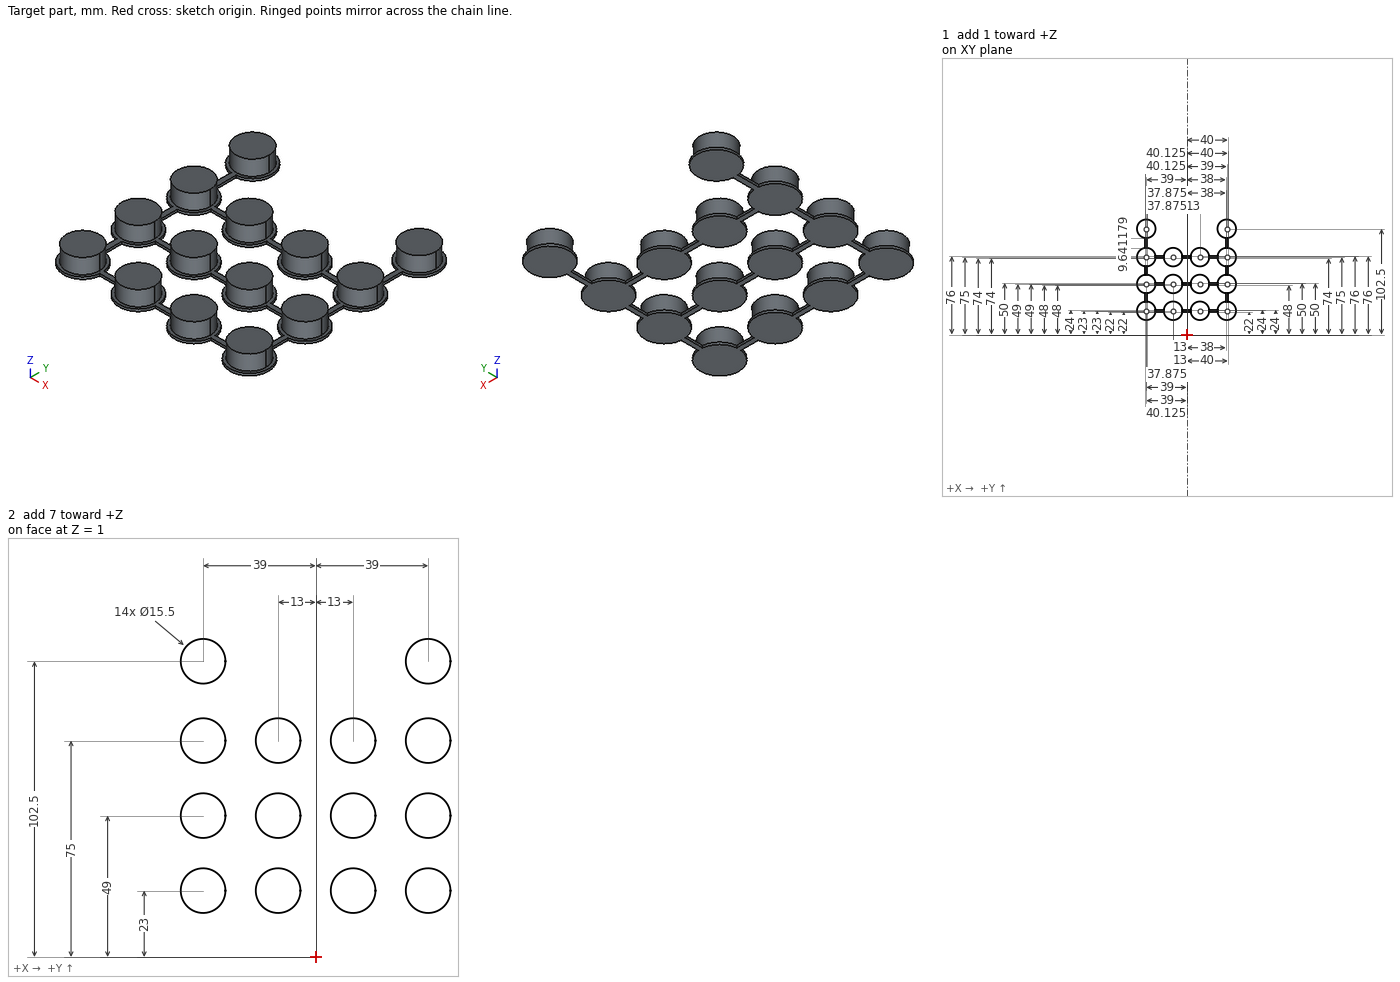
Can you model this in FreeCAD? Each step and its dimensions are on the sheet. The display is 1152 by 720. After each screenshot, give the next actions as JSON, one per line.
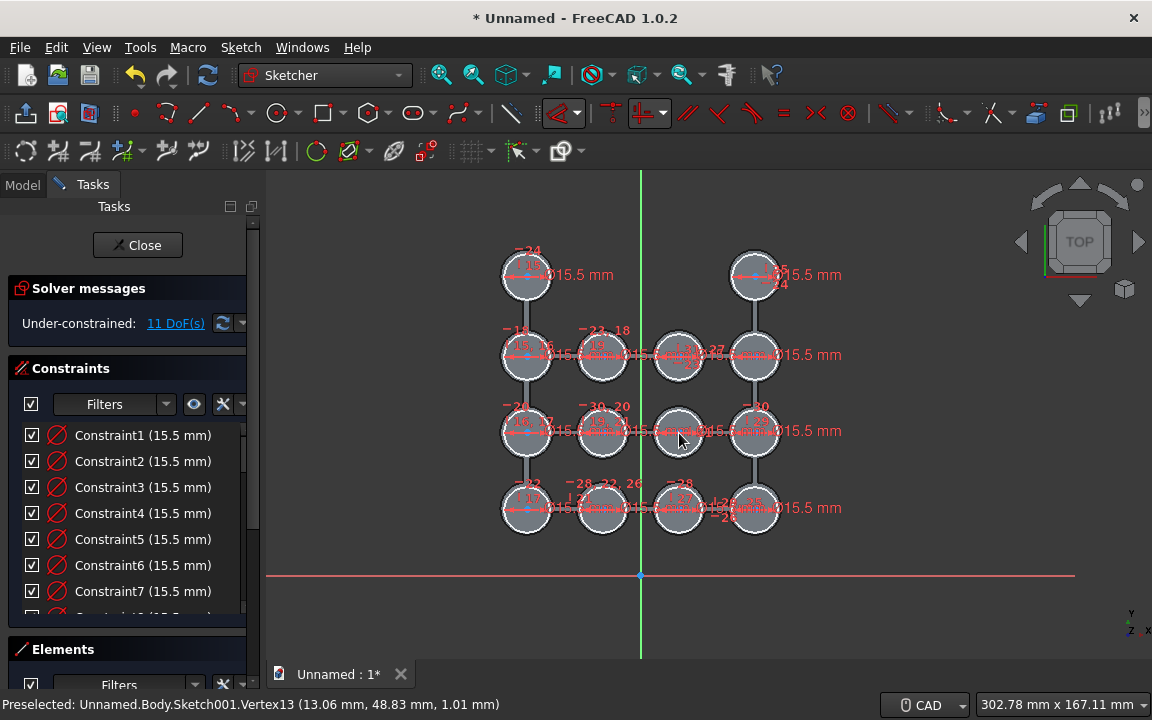
{"action": "left_click", "coordinate": [603, 433]}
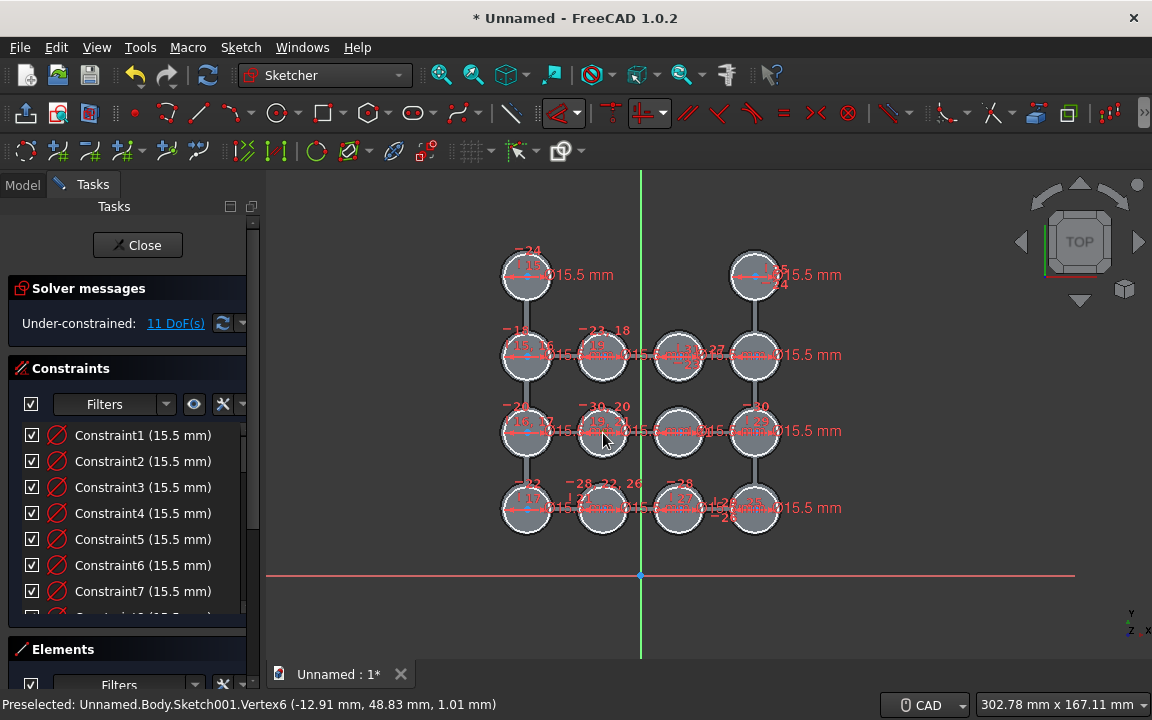
{"action": "left_click", "coordinate": [679, 433]}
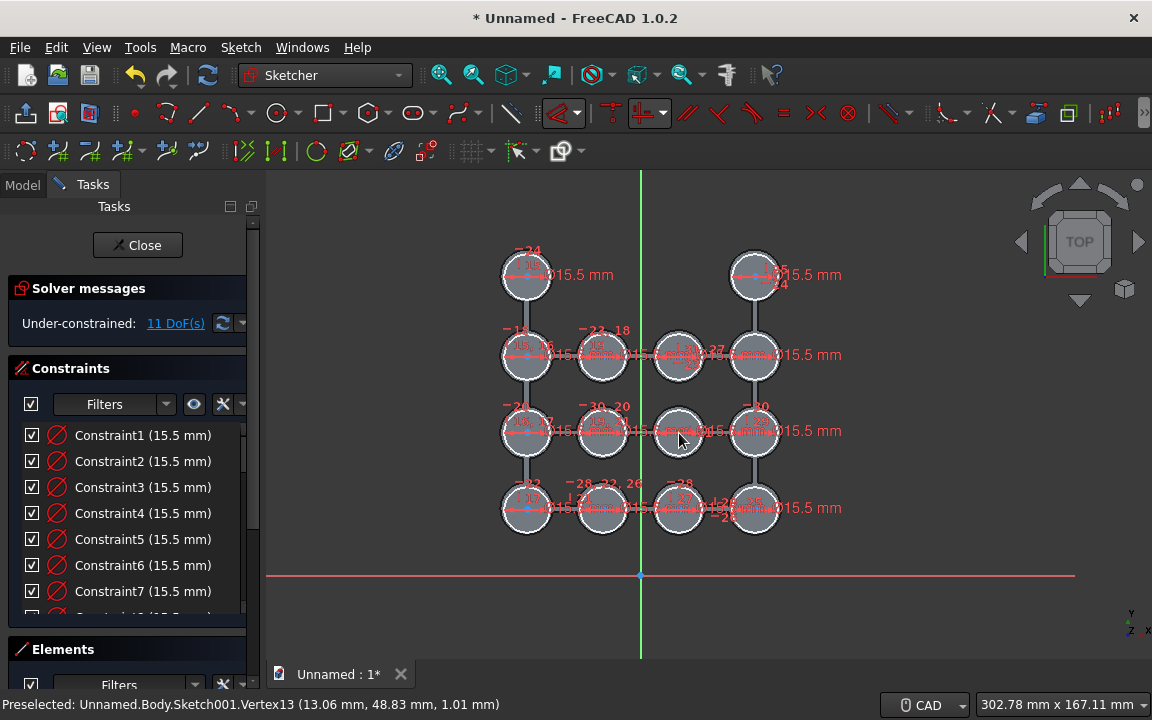
{"action": "left_click", "coordinate": [666, 114]}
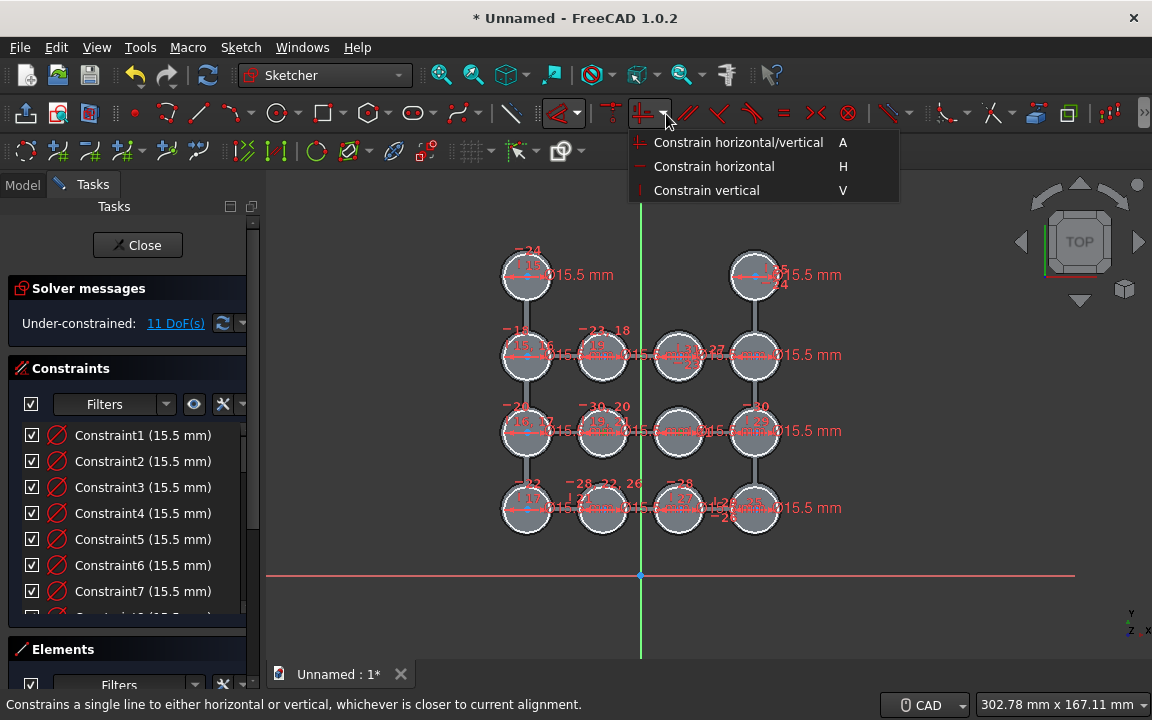
{"action": "left_click", "coordinate": [764, 166]}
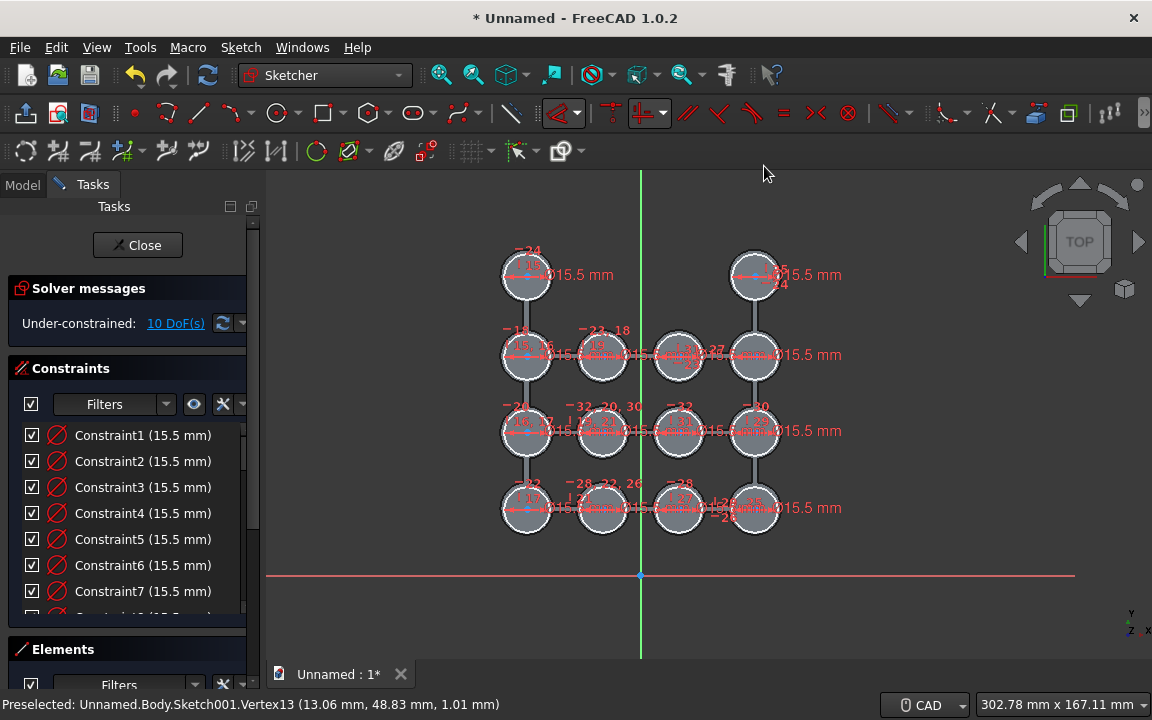
{"action": "left_click", "coordinate": [755, 433]}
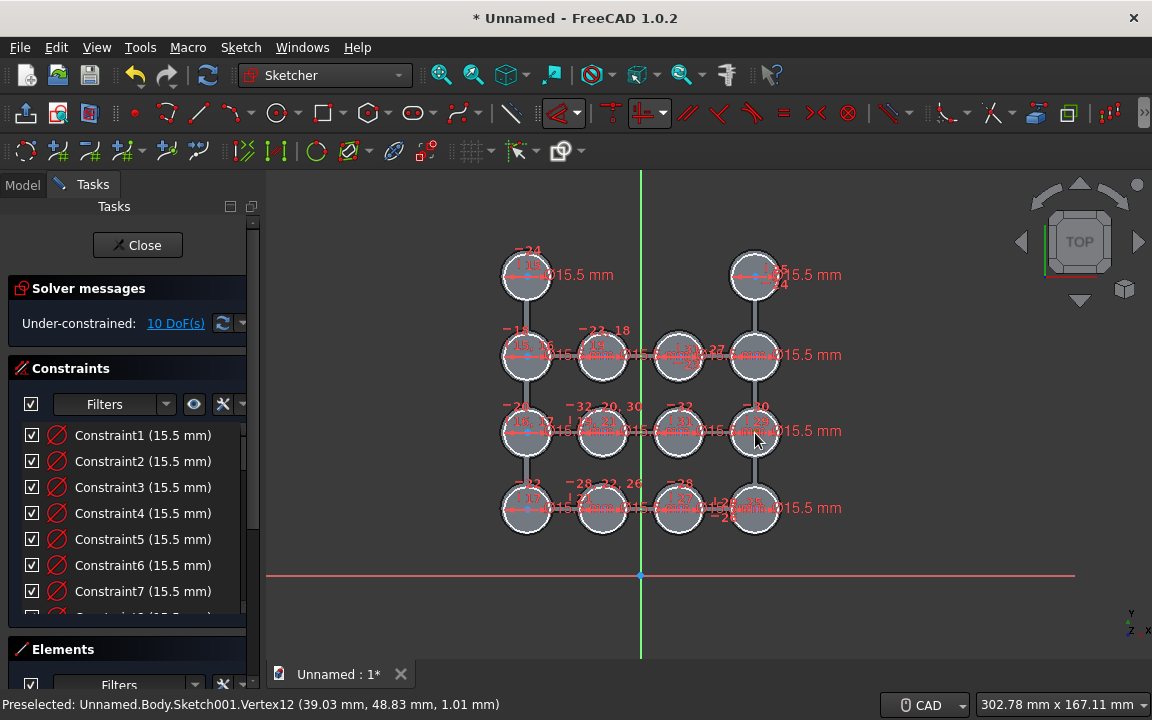
{"action": "left_click", "coordinate": [755, 357]}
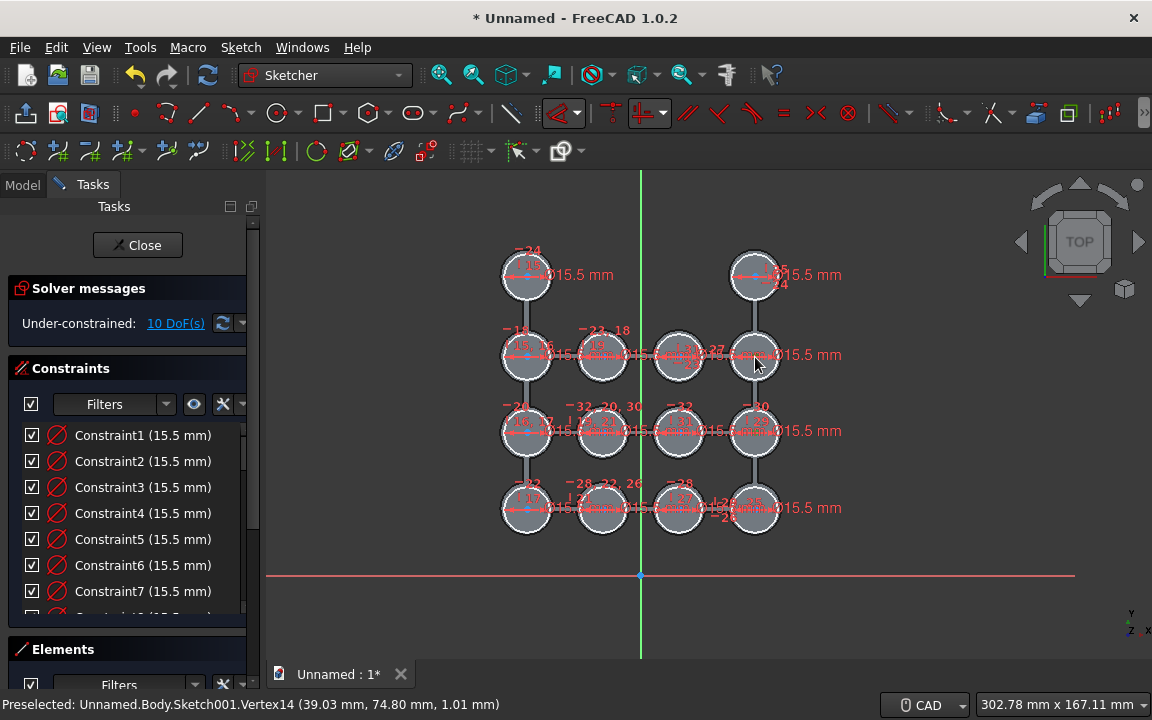
{"action": "key", "text": "v"}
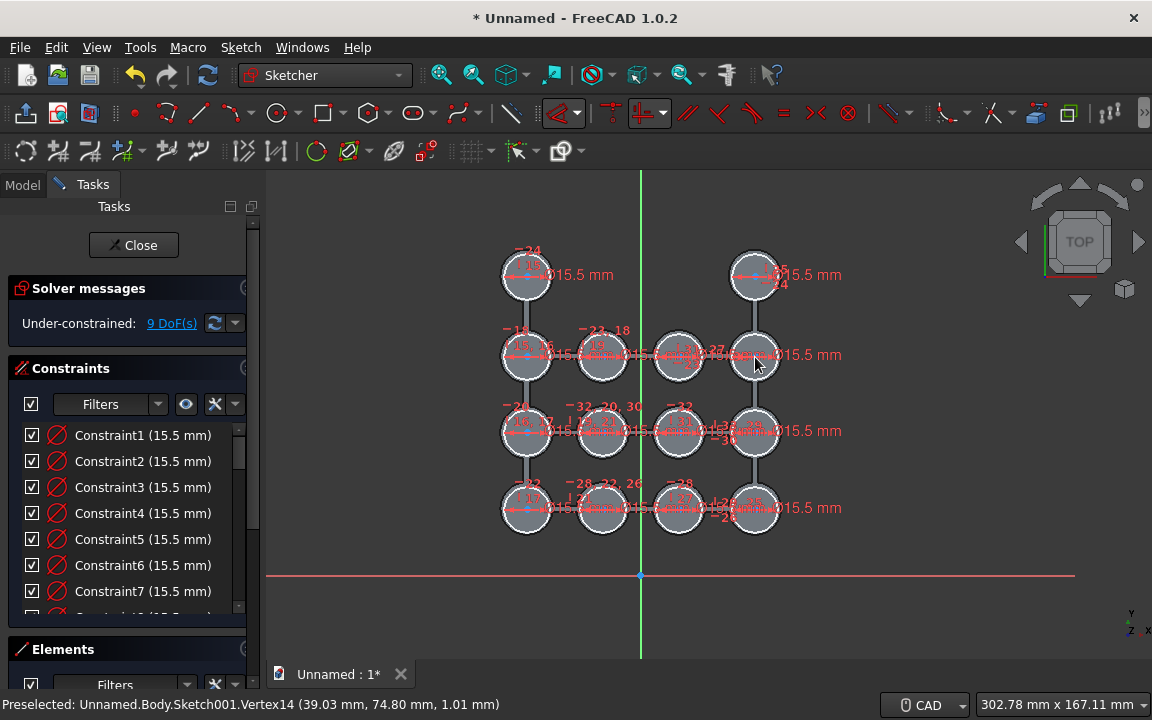
{"action": "left_click", "coordinate": [679, 357]}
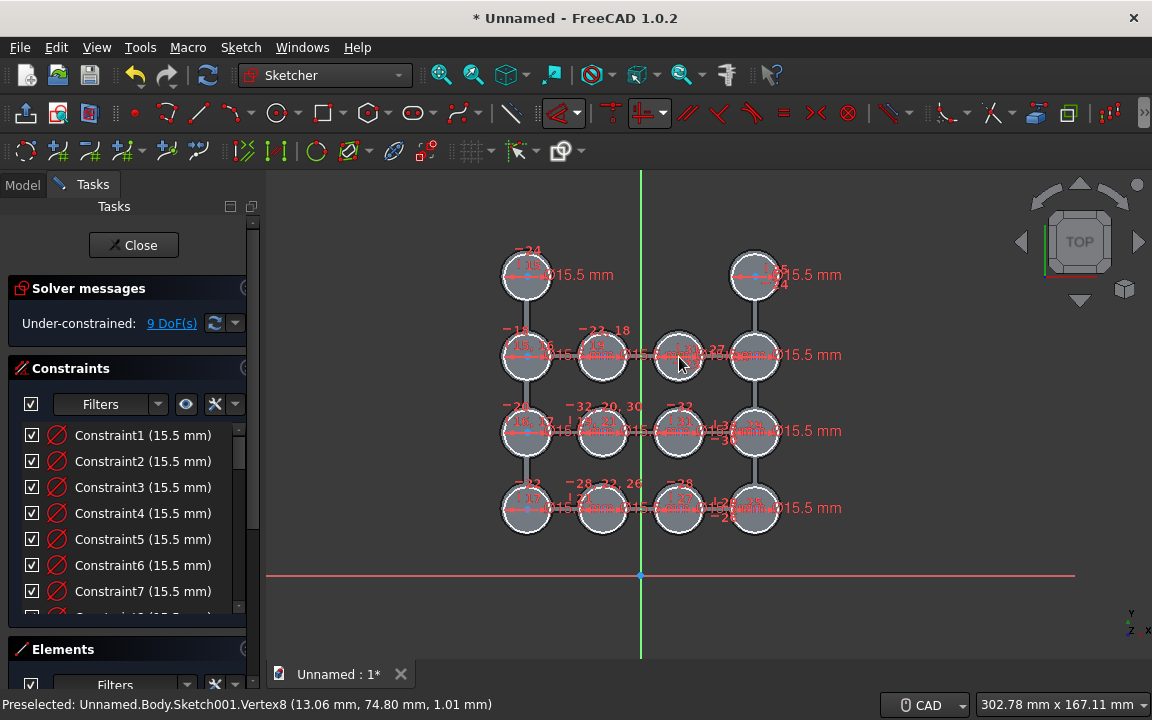
{"action": "left_click", "coordinate": [755, 357]}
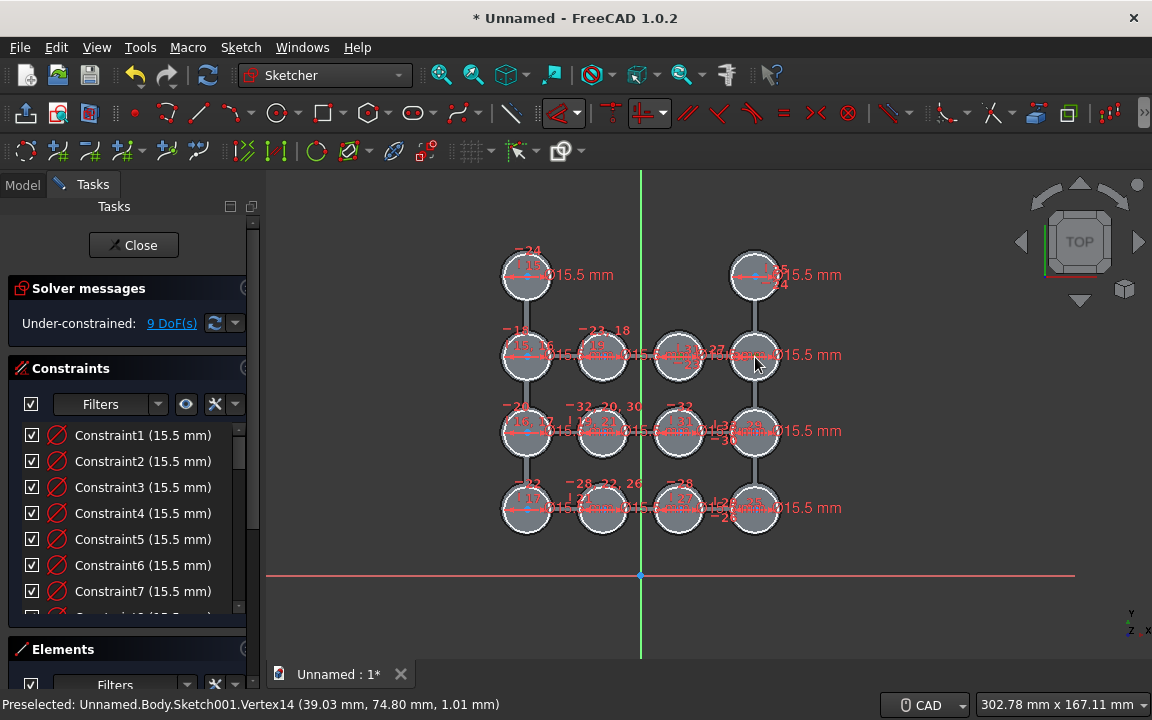
{"action": "key", "text": "h"}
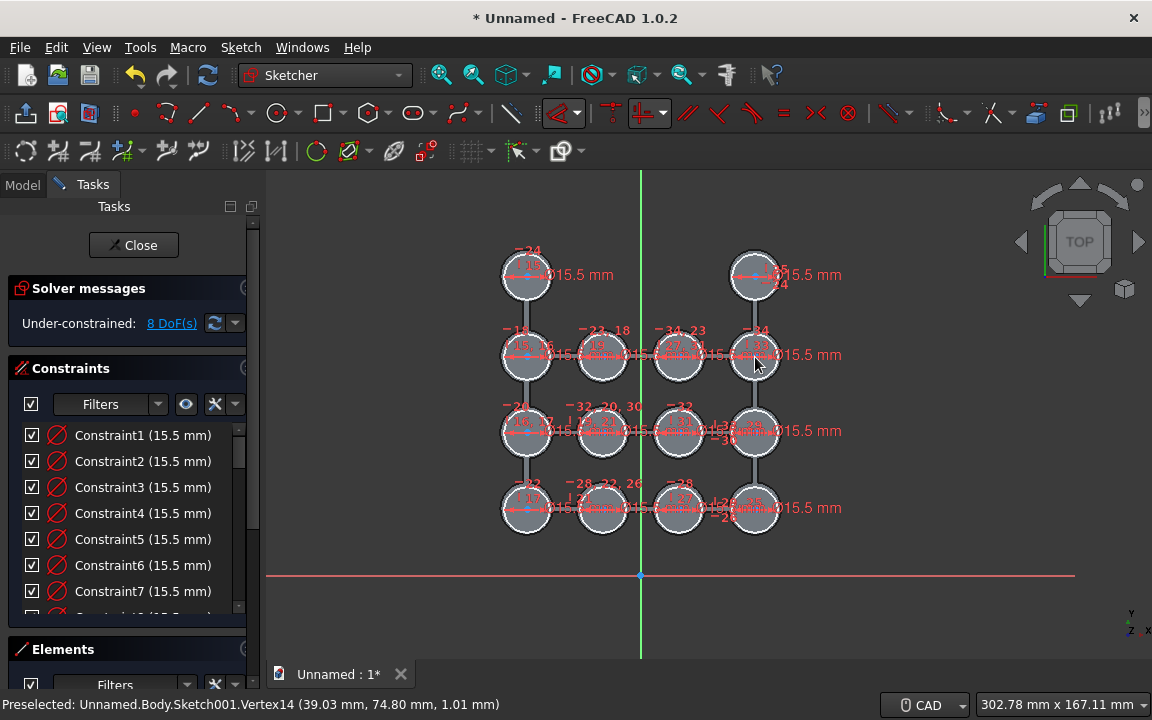
{"action": "left_click", "coordinate": [527, 277]}